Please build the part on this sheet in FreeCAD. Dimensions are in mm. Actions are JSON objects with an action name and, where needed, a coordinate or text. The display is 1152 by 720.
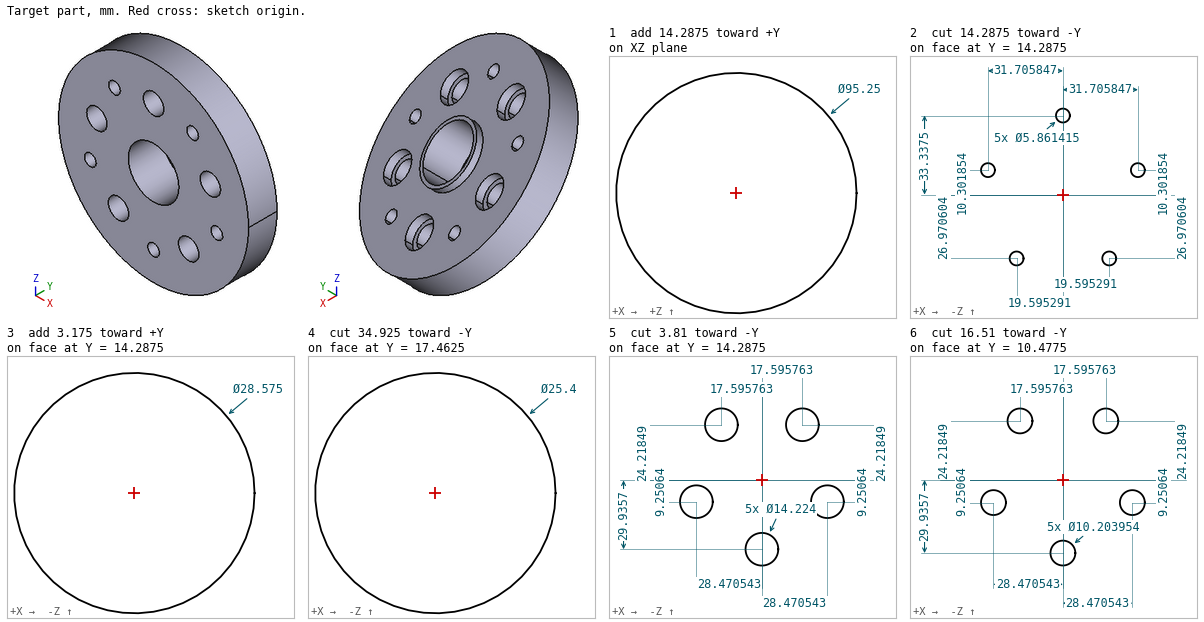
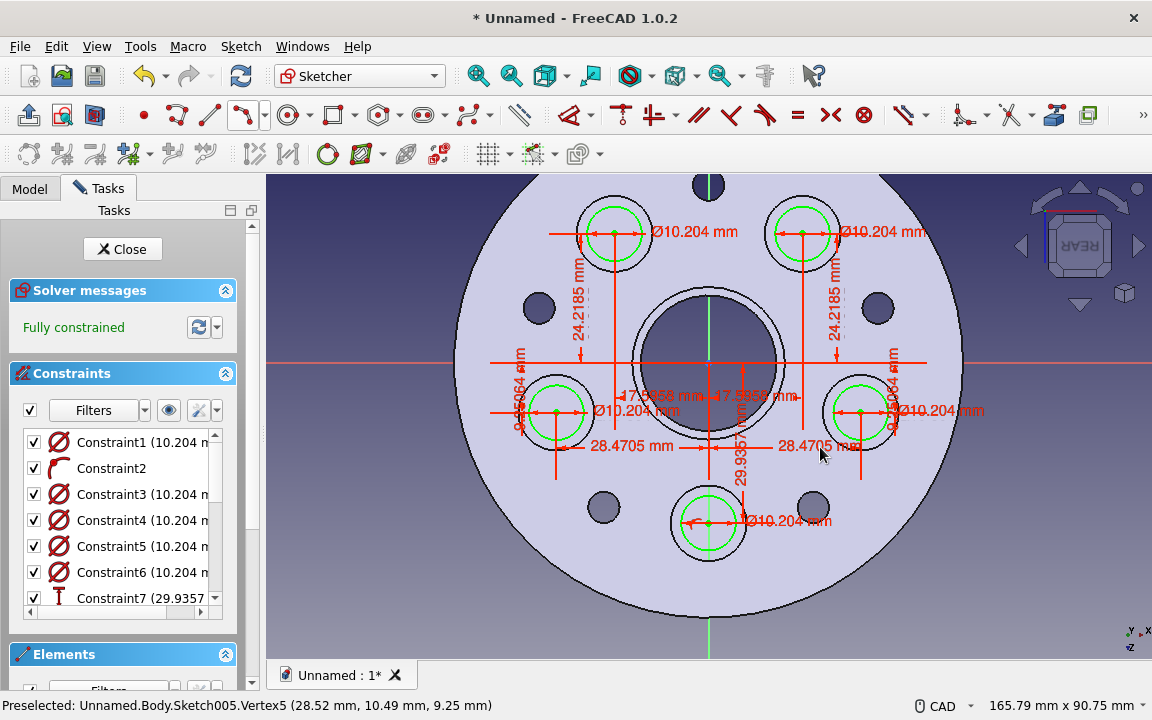
{"action": "left_click", "coordinate": [123, 249]}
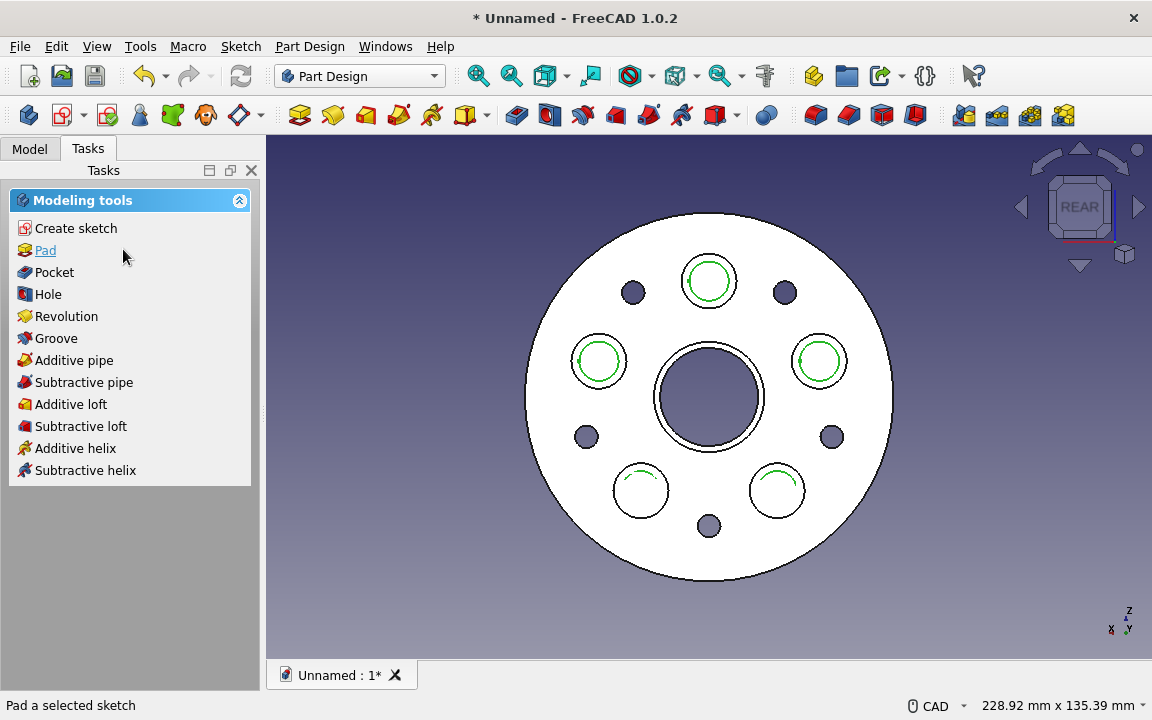
{"action": "left_click", "coordinate": [517, 116]}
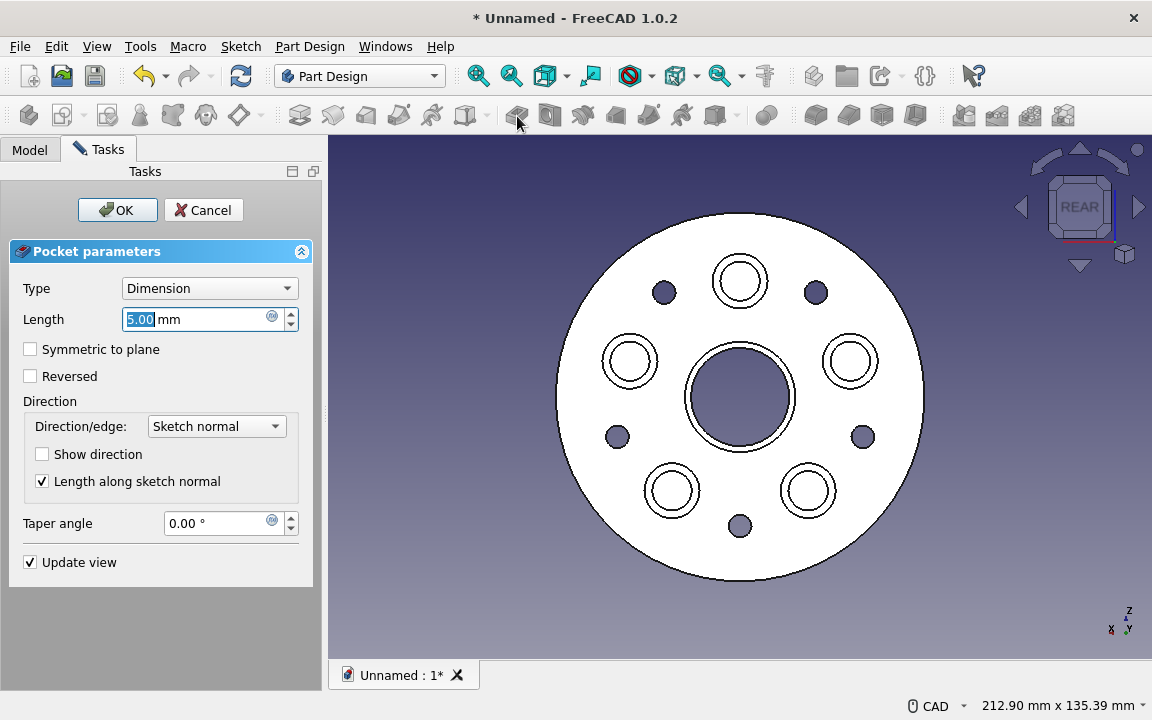
{"action": "type", "text": "16.51"}
{"action": "key", "text": "Tab"}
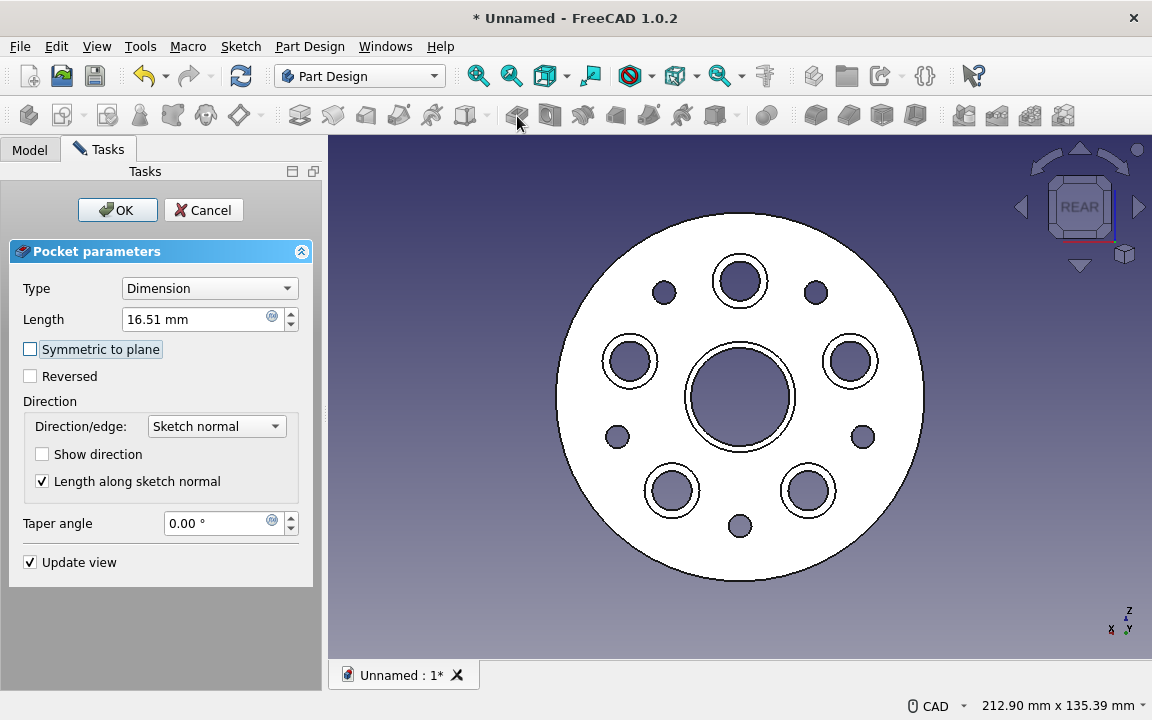
{"action": "left_click", "coordinate": [118, 210]}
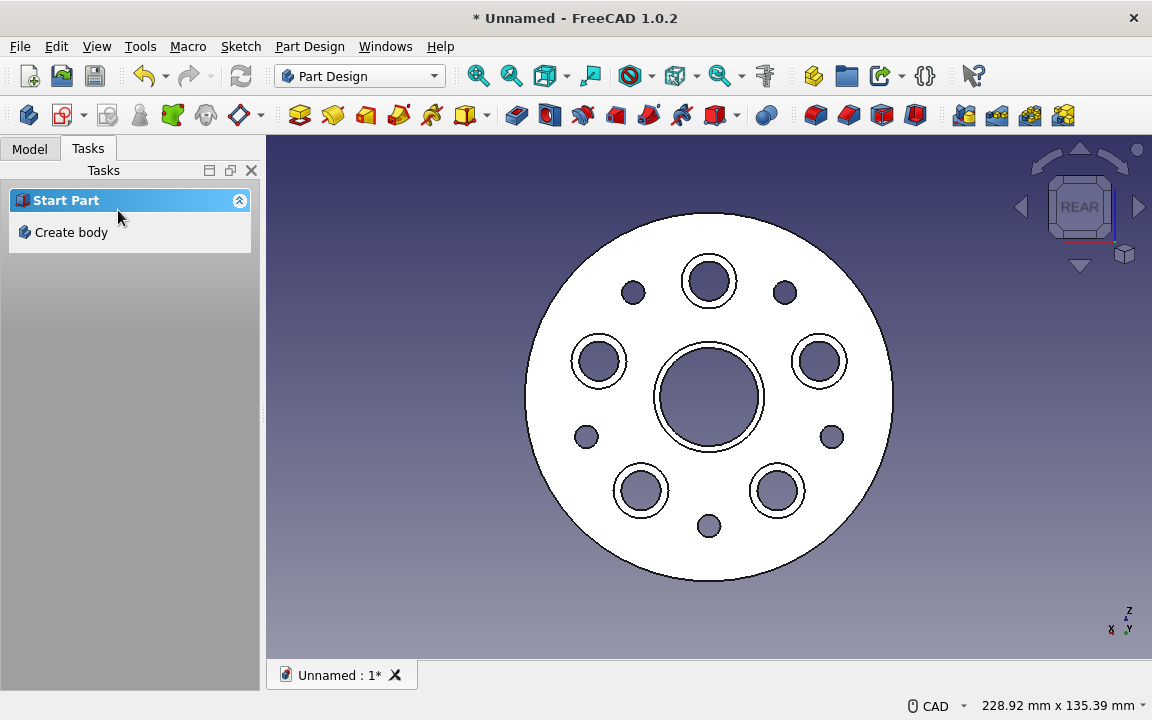
{"action": "key", "text": "0"}